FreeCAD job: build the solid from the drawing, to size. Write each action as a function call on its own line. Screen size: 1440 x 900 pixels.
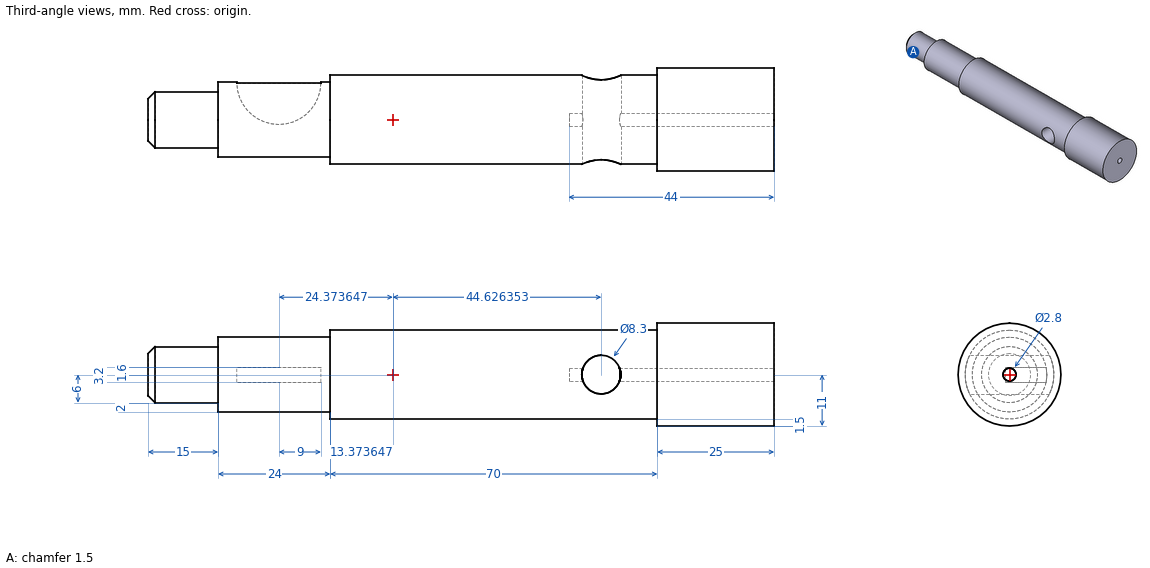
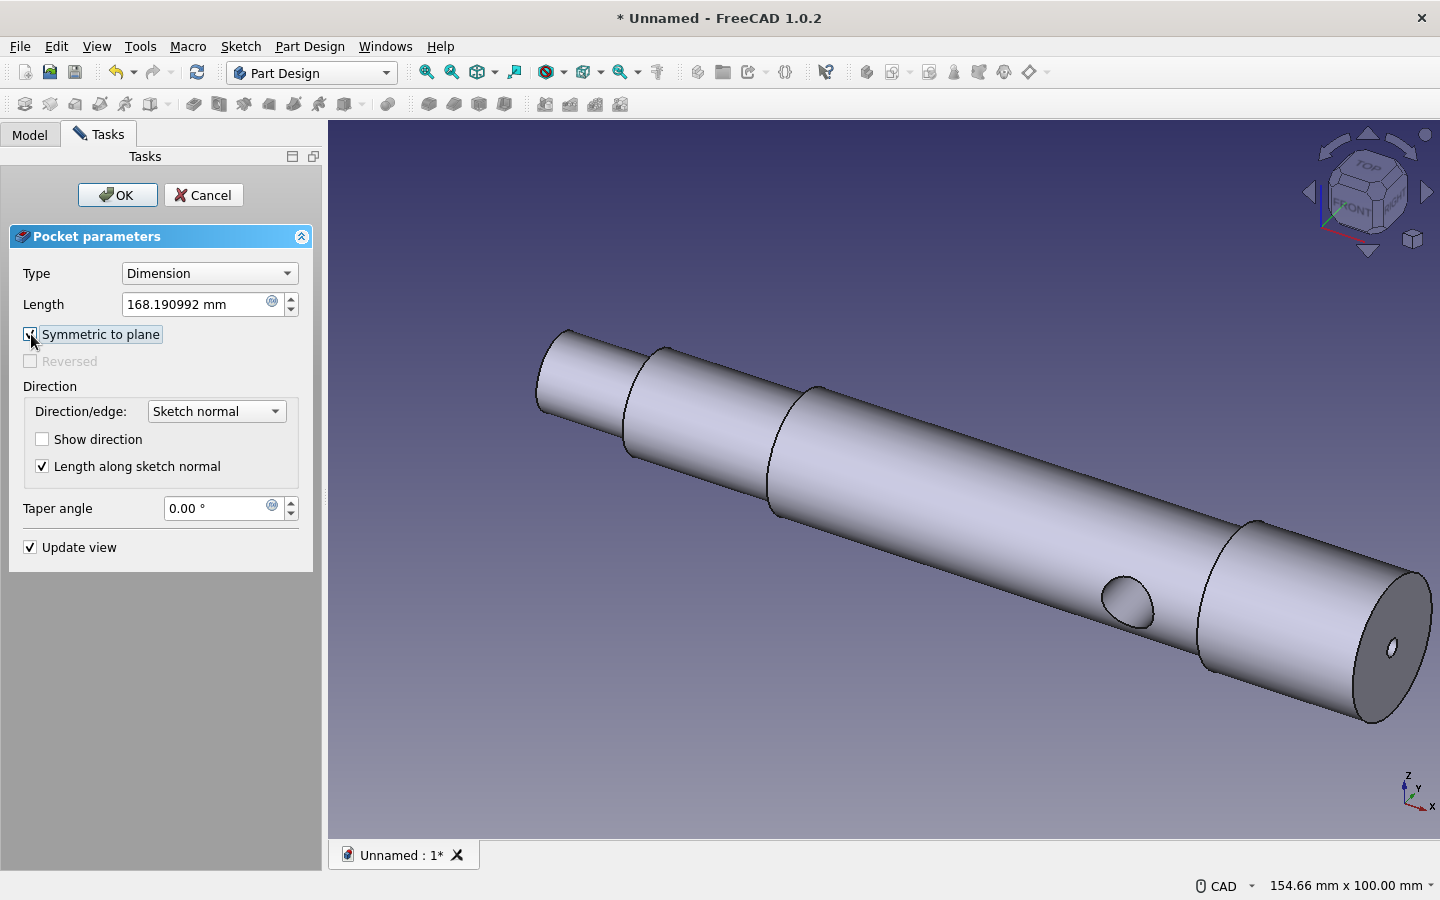
click(118, 195)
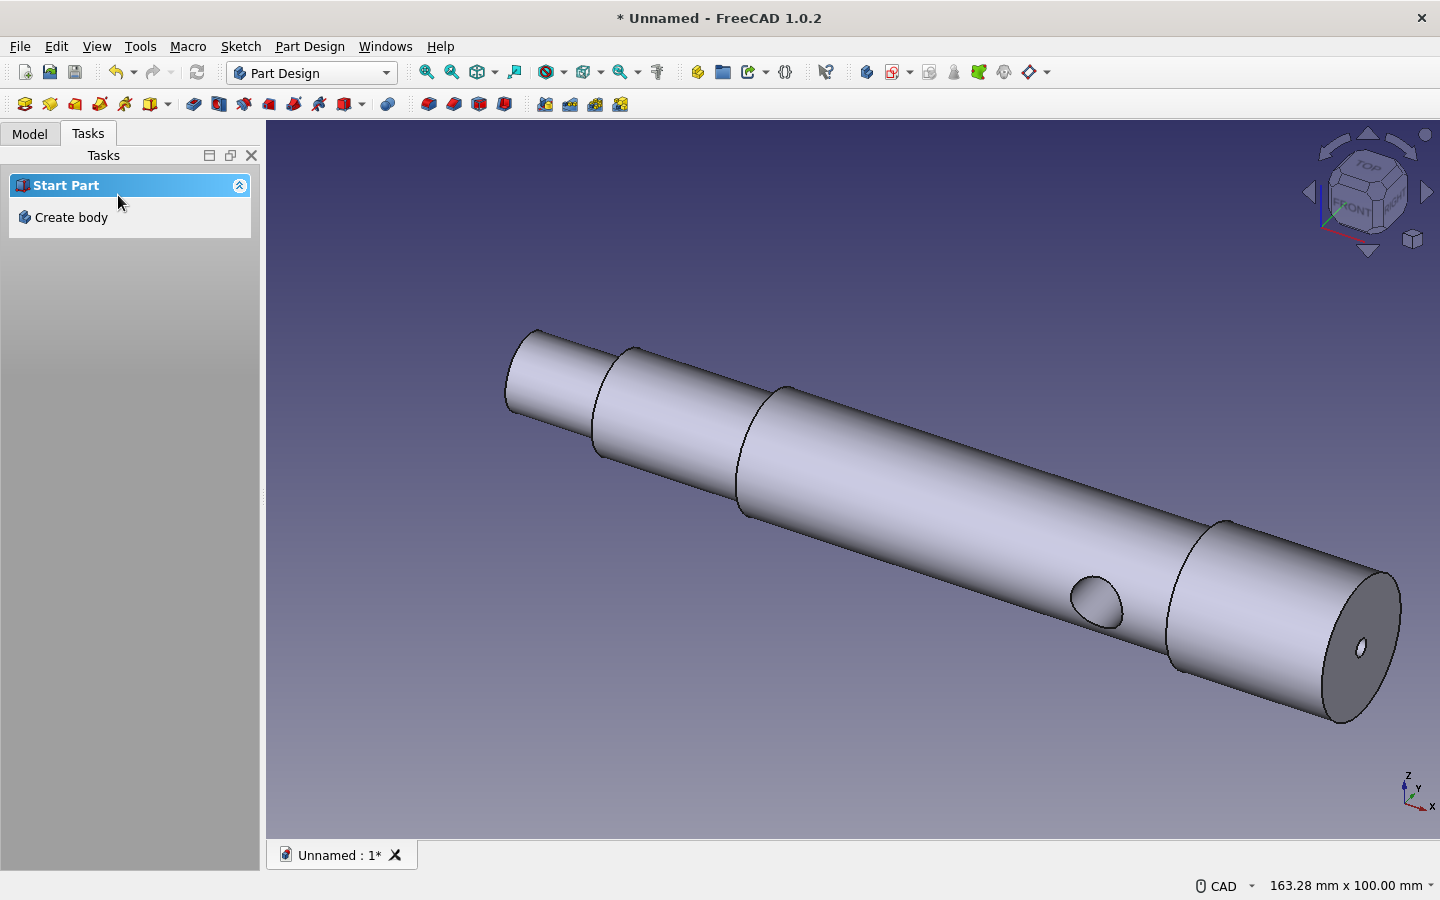
click(30, 134)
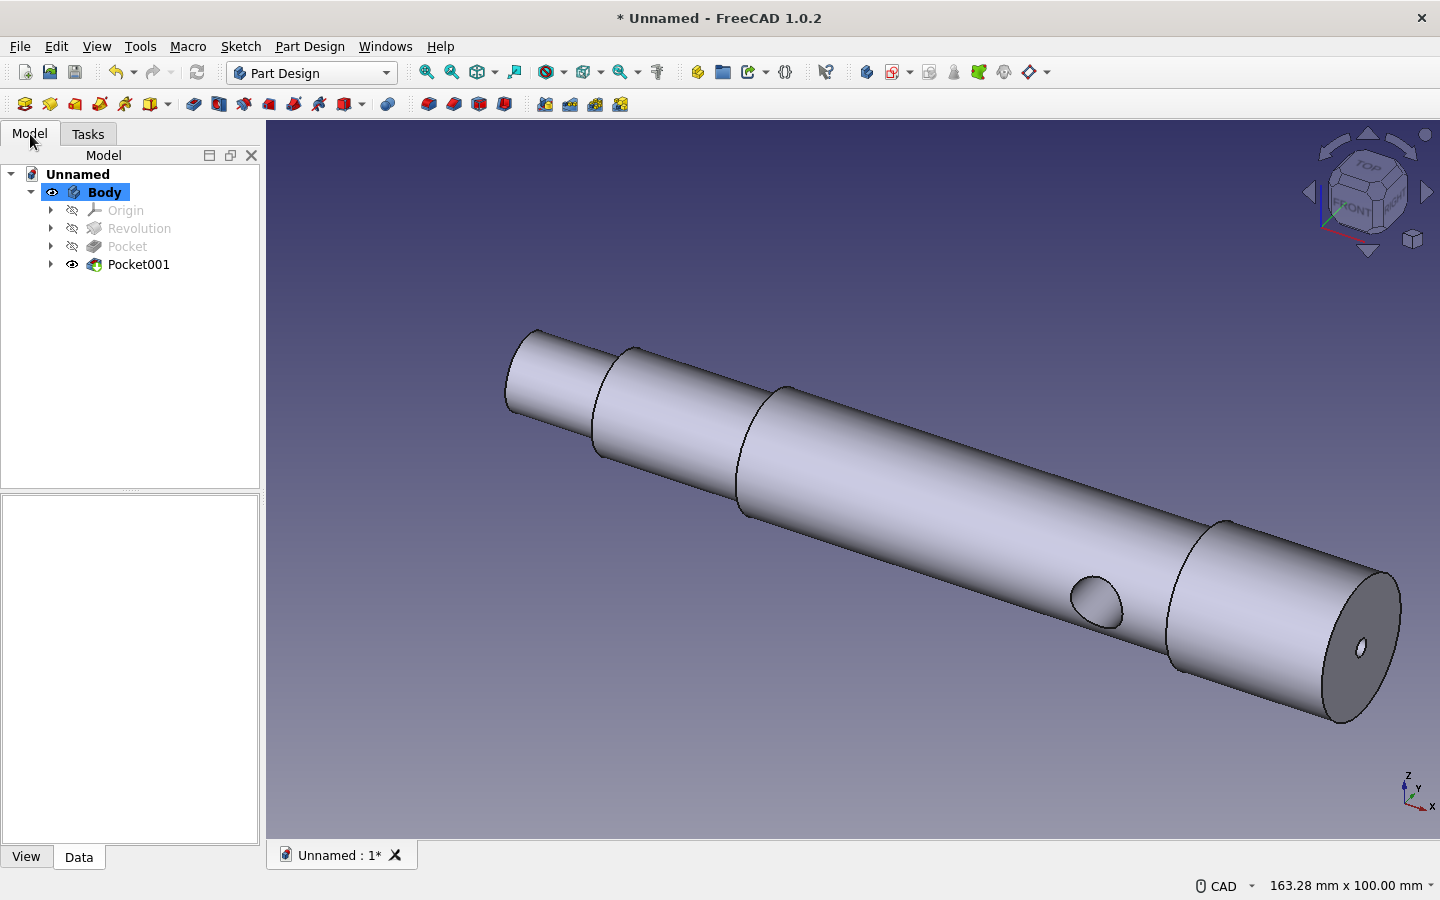
click(51, 210)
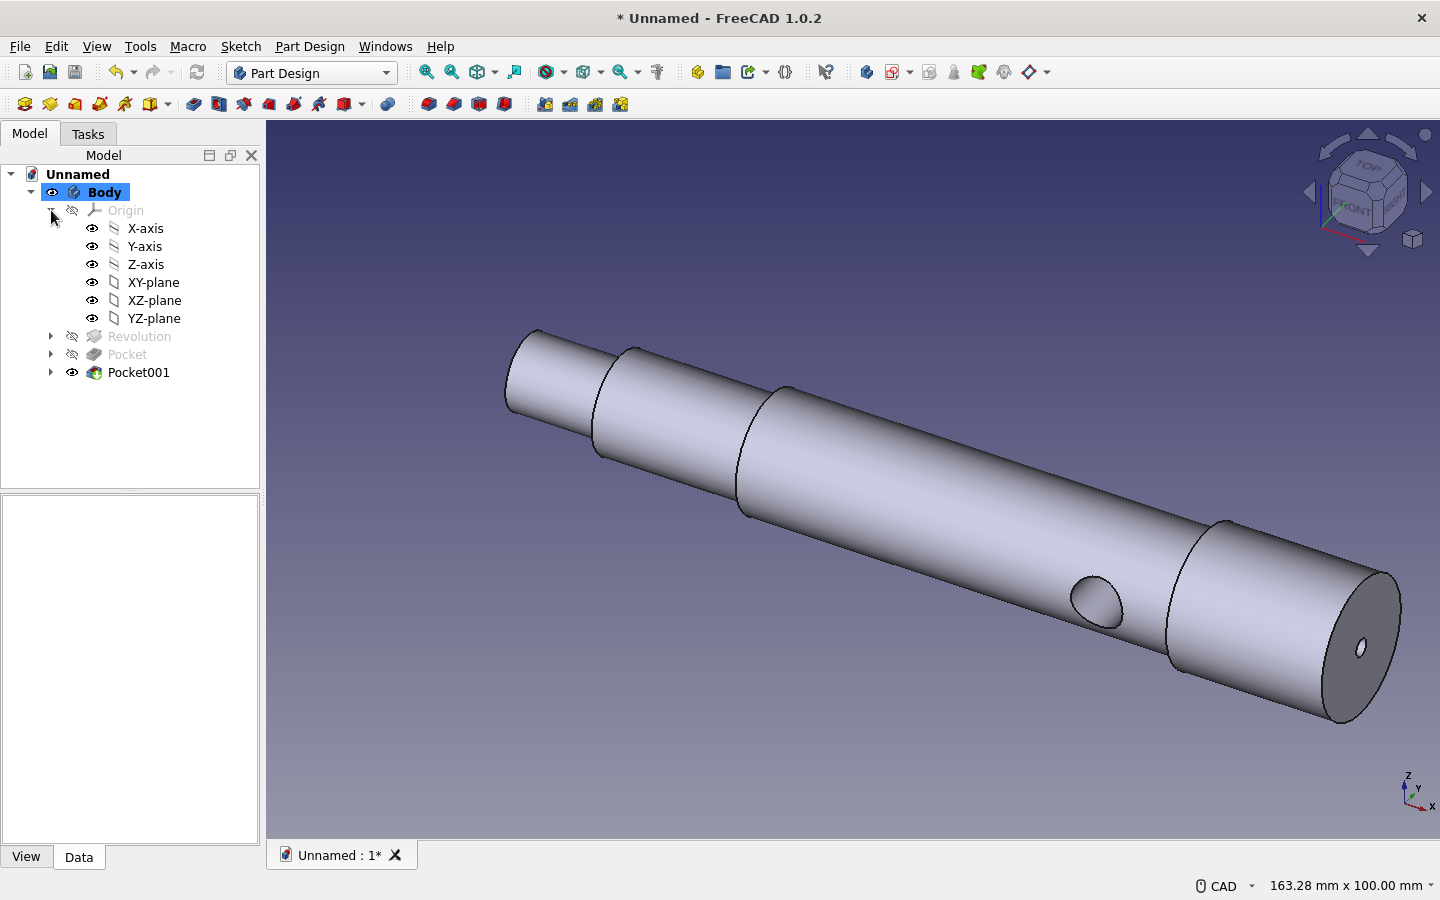
click(137, 300)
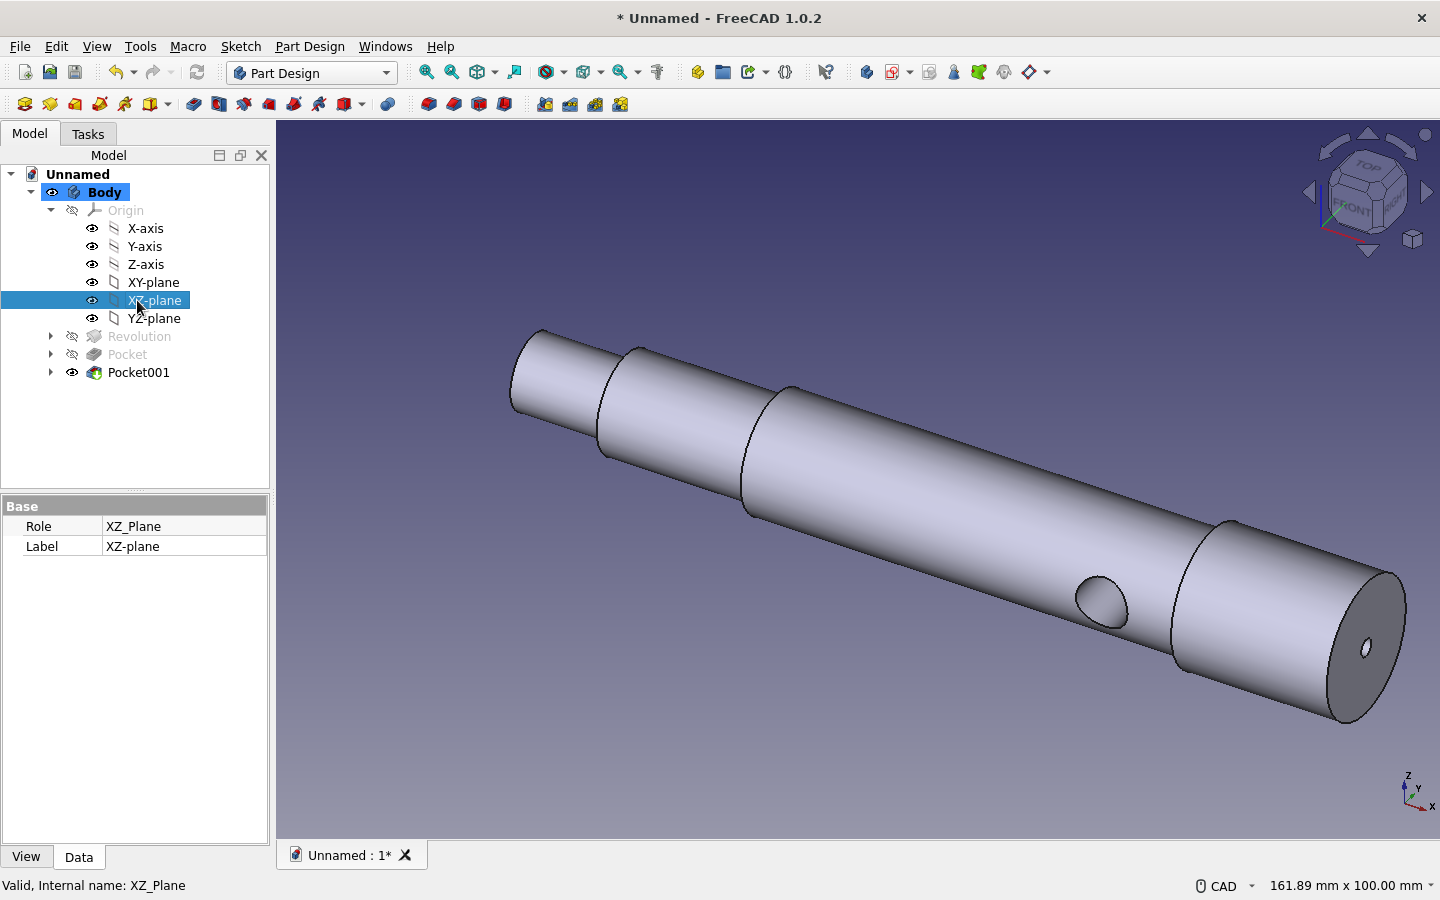
click(1028, 72)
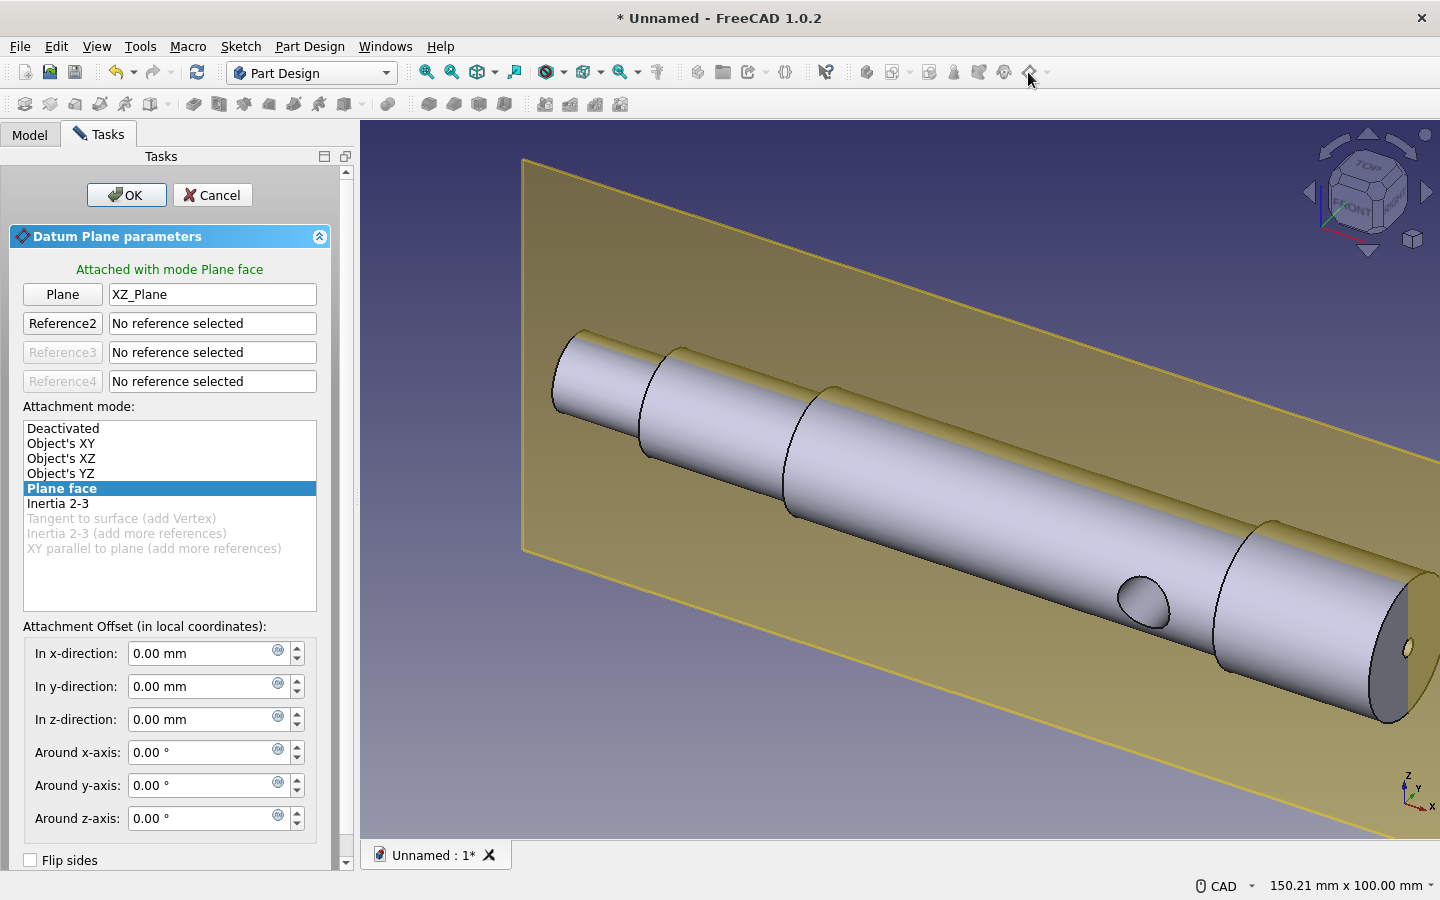
triple_click(210, 720)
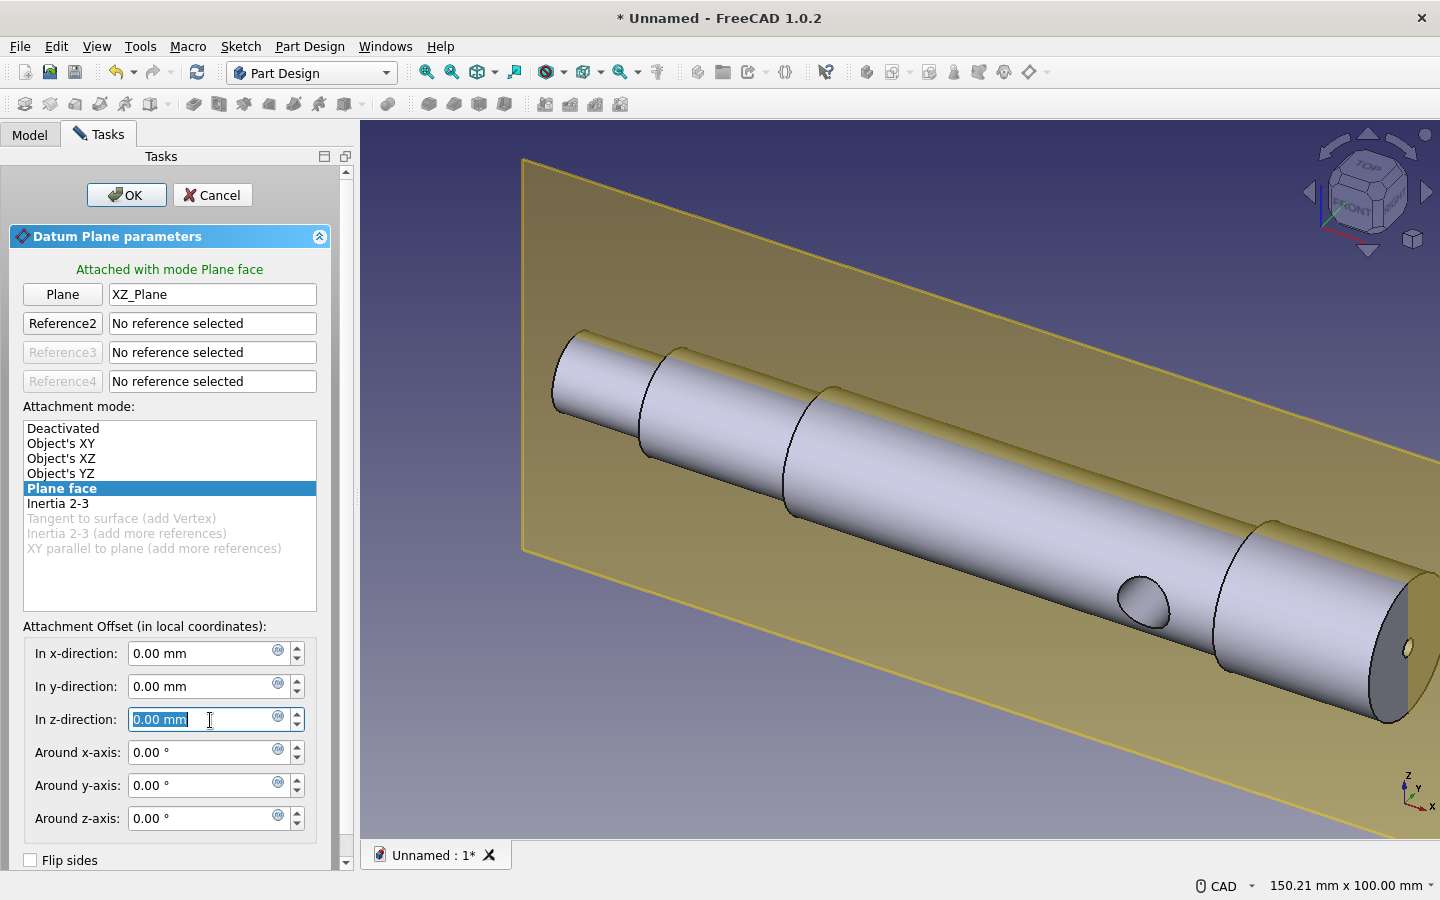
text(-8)
key(Tab)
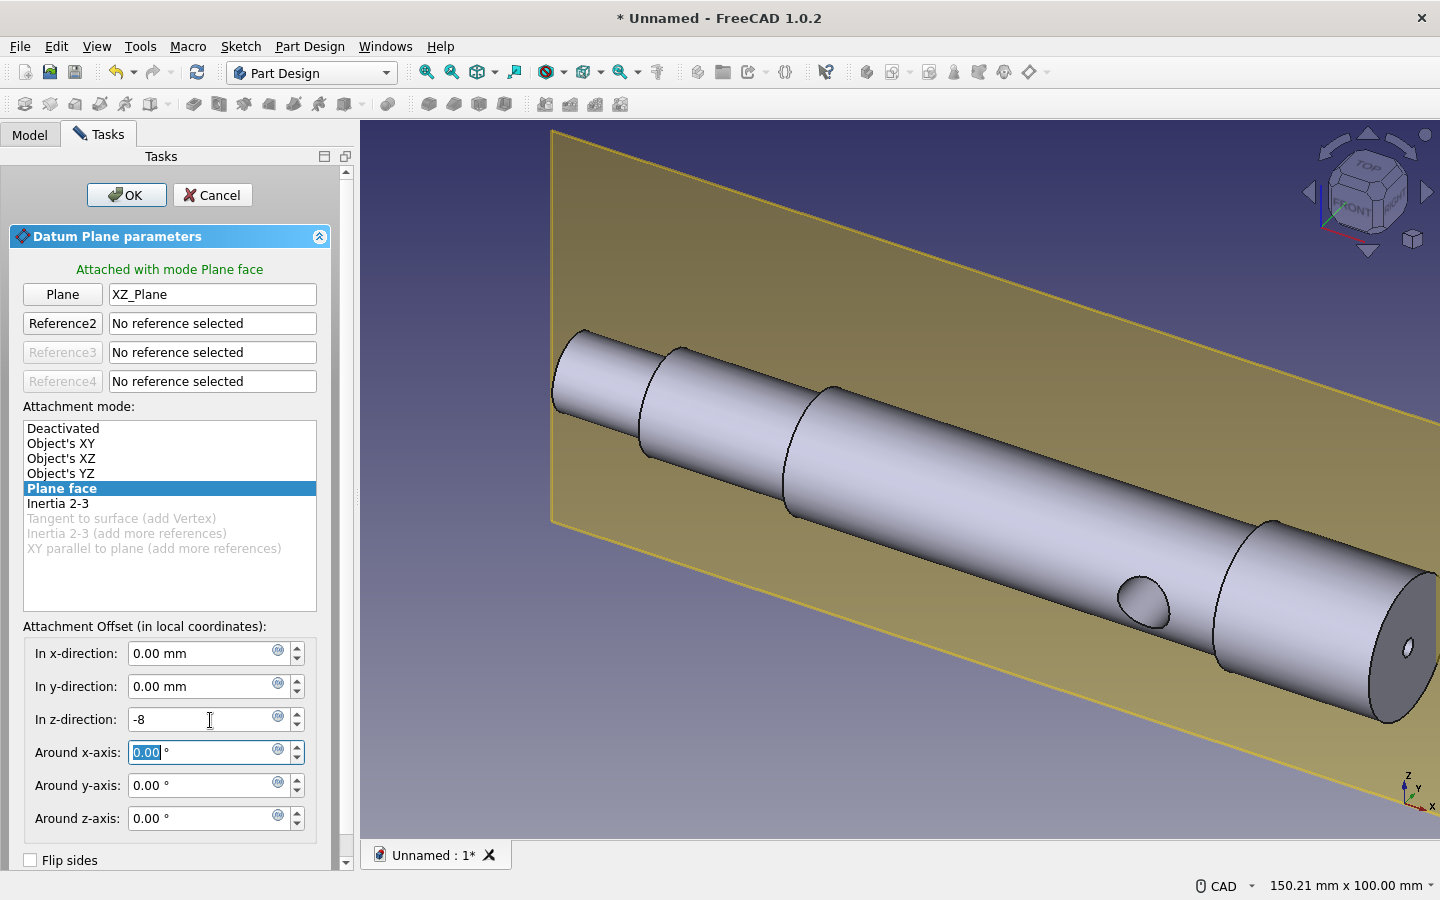
click(127, 195)